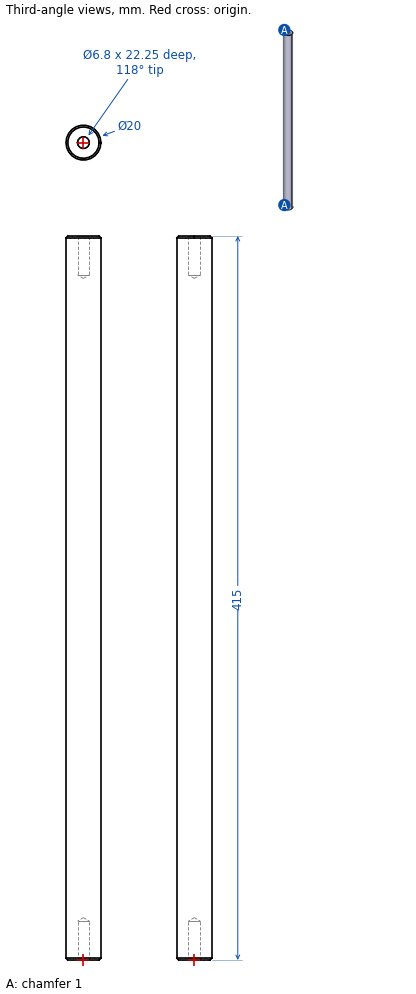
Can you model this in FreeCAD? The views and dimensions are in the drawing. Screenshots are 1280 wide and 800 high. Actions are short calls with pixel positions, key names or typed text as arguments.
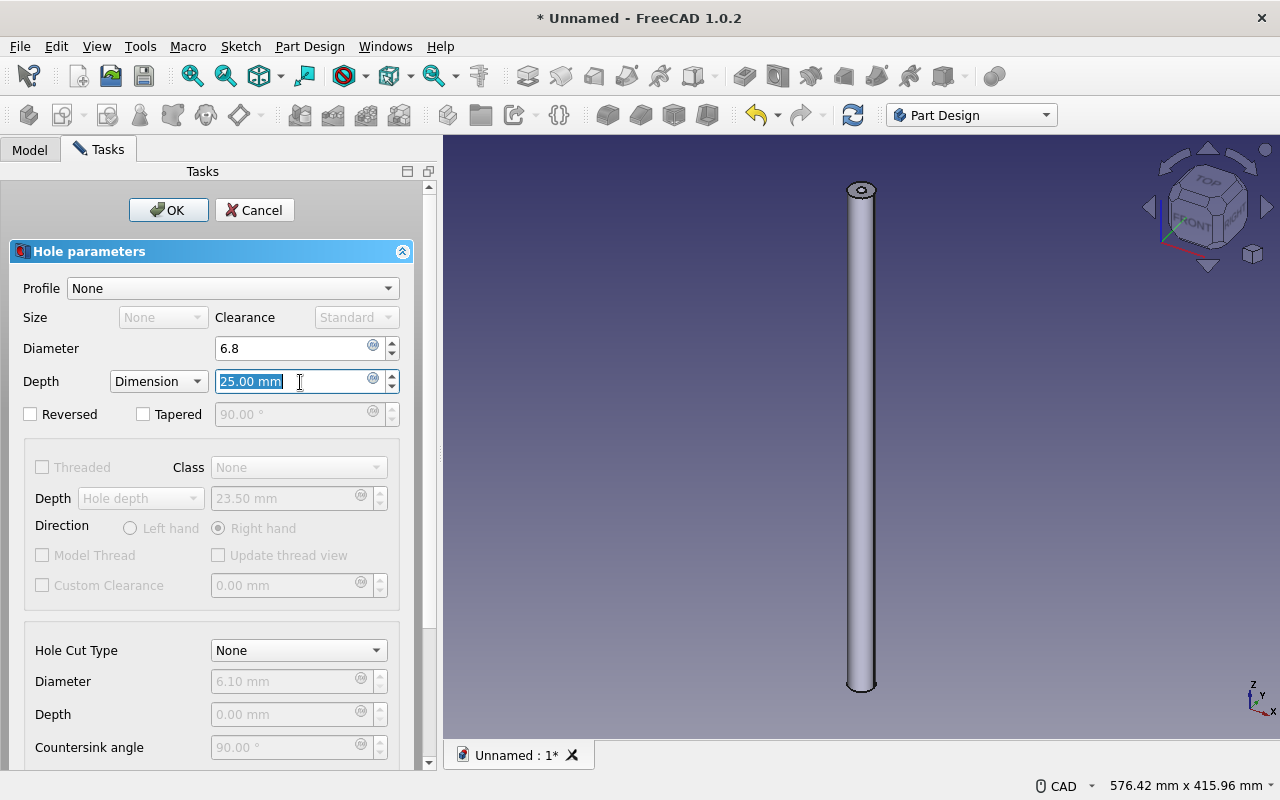
text(22.25)
key(Tab)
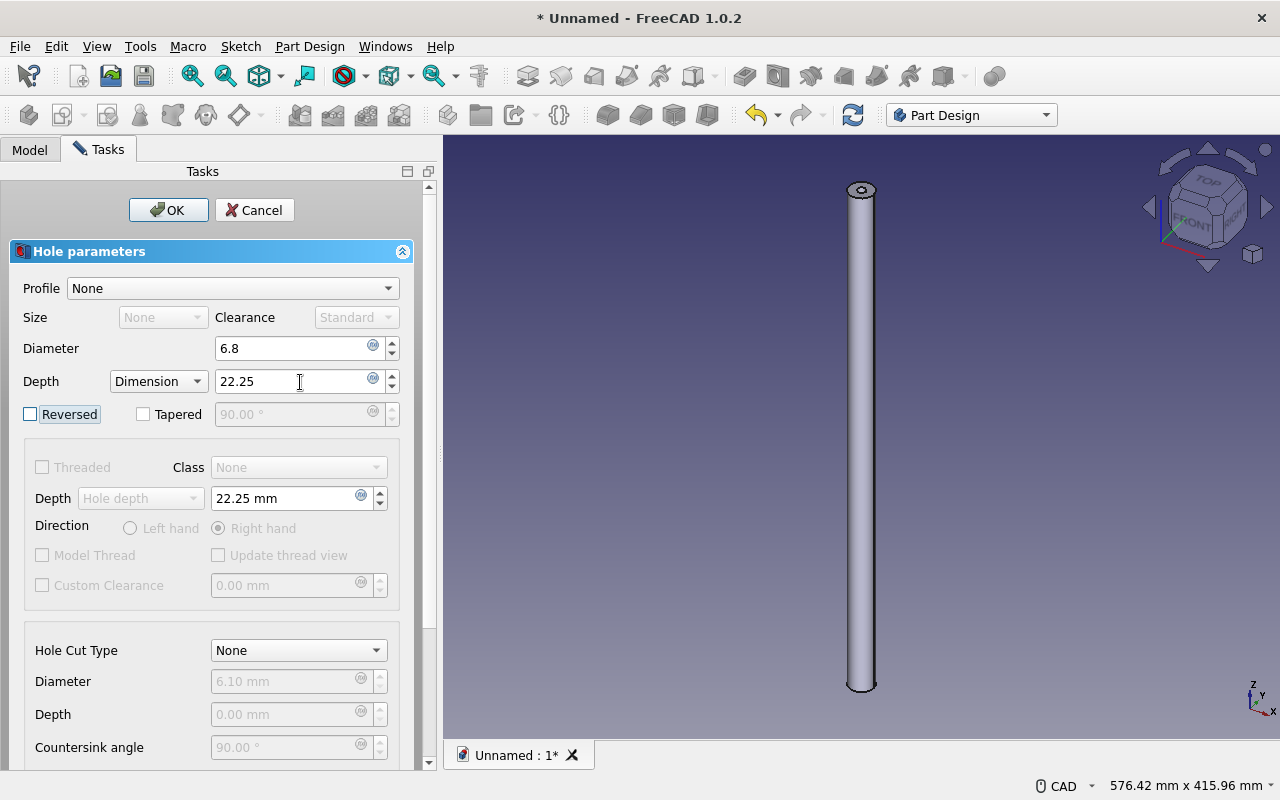
click(169, 210)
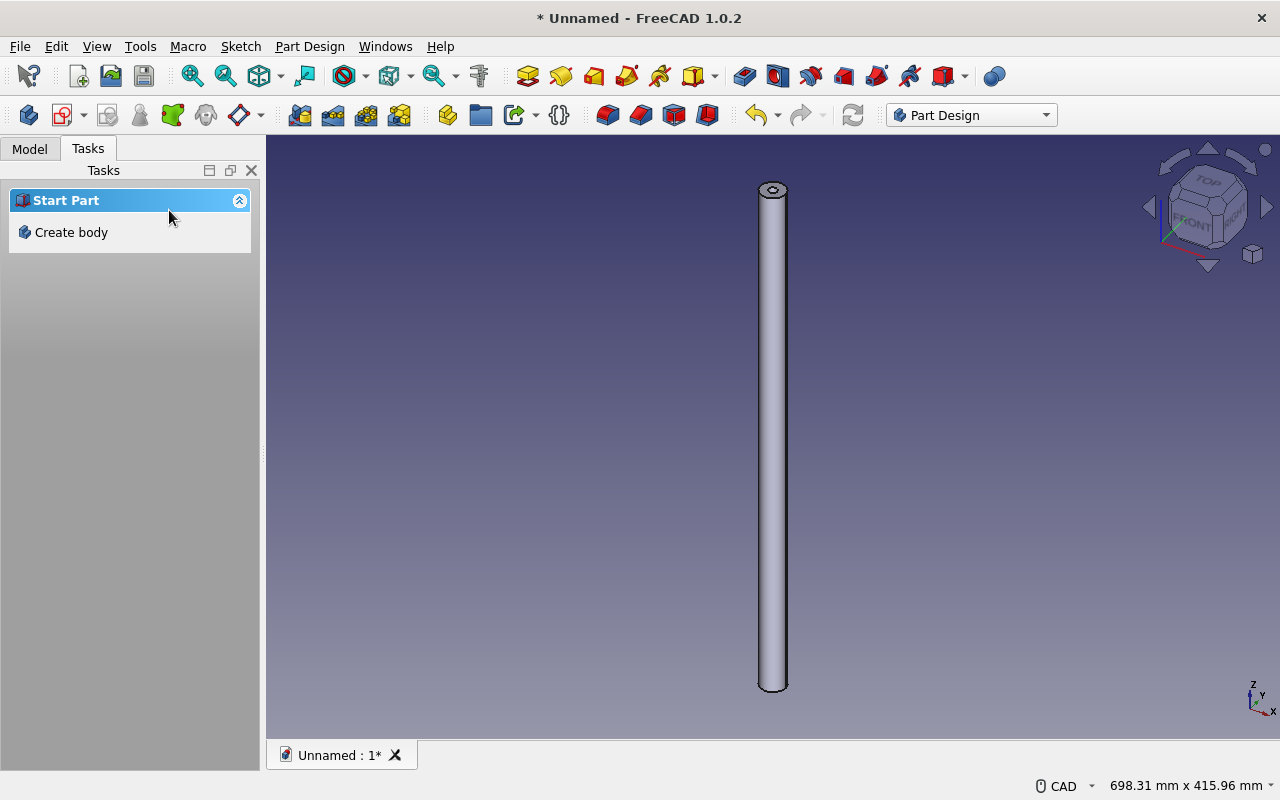
click(760, 185)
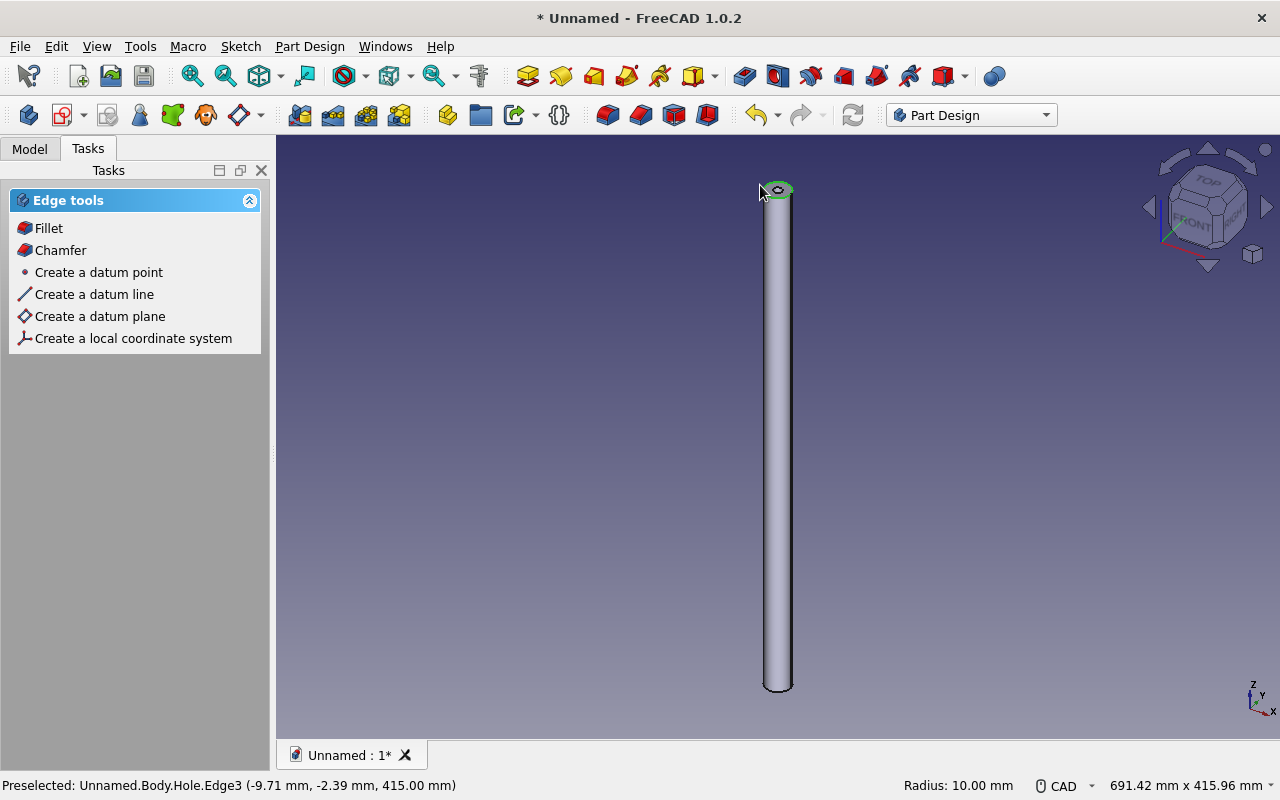
key(0)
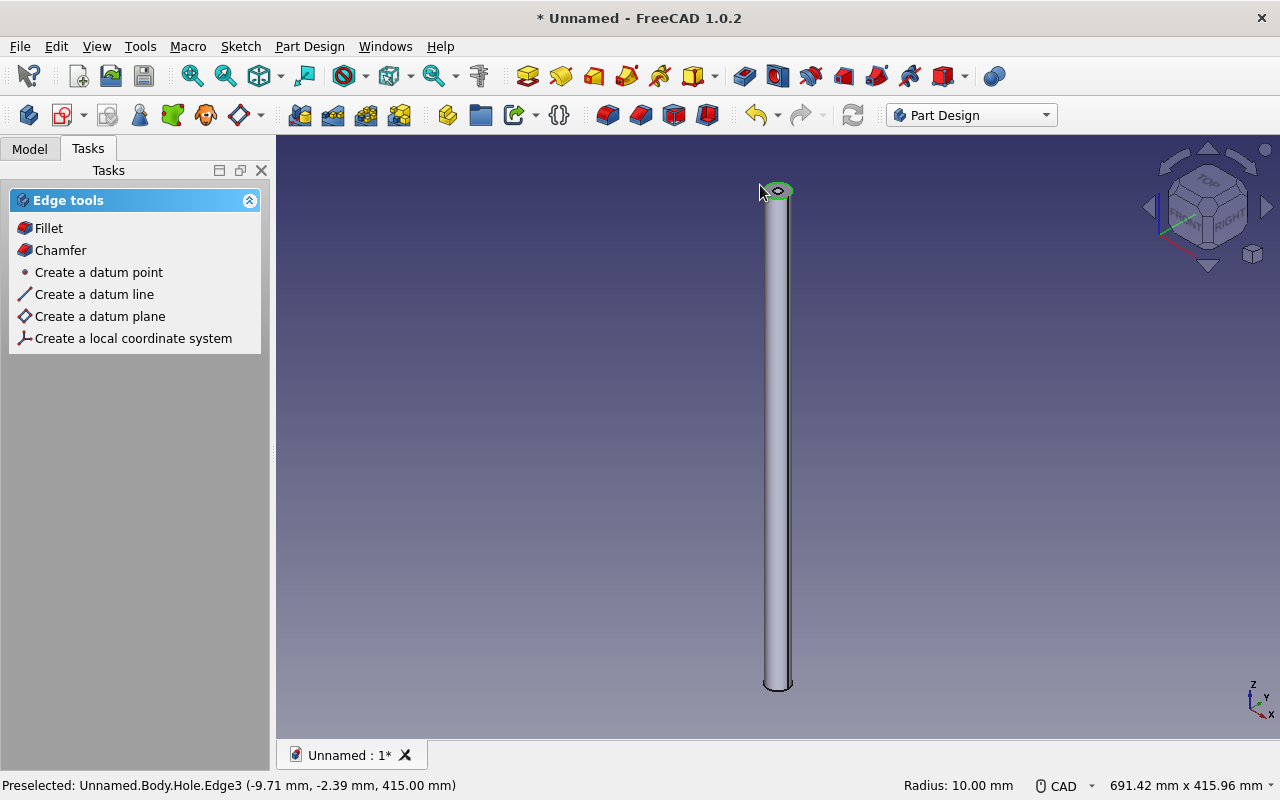
key(2)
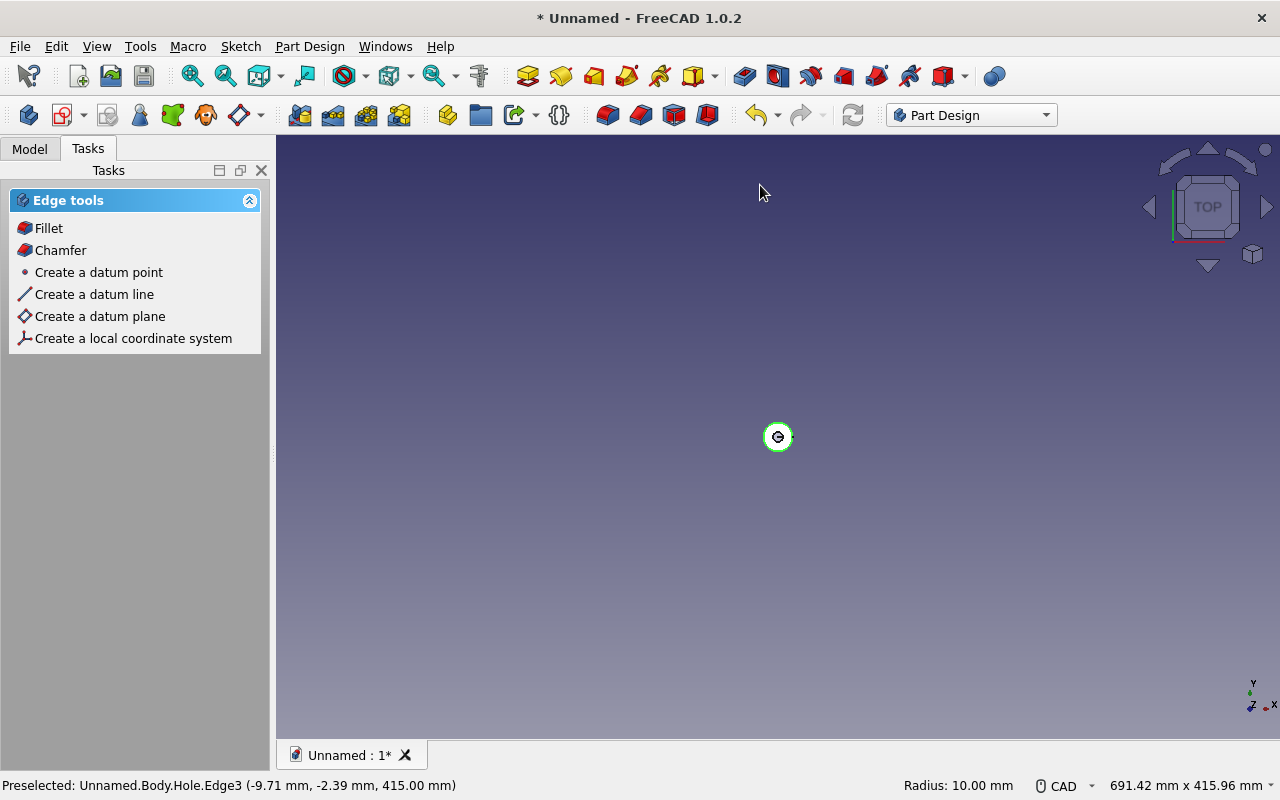
click(193, 76)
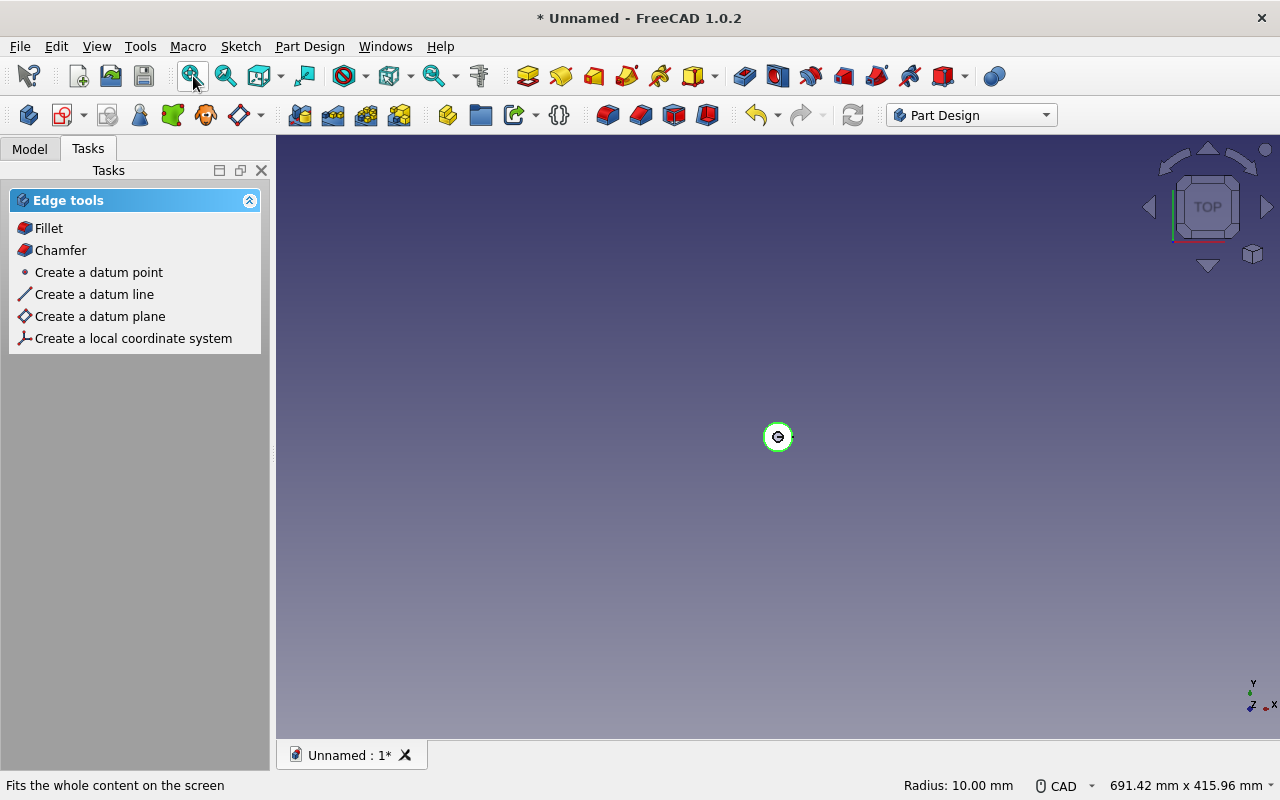
key(1)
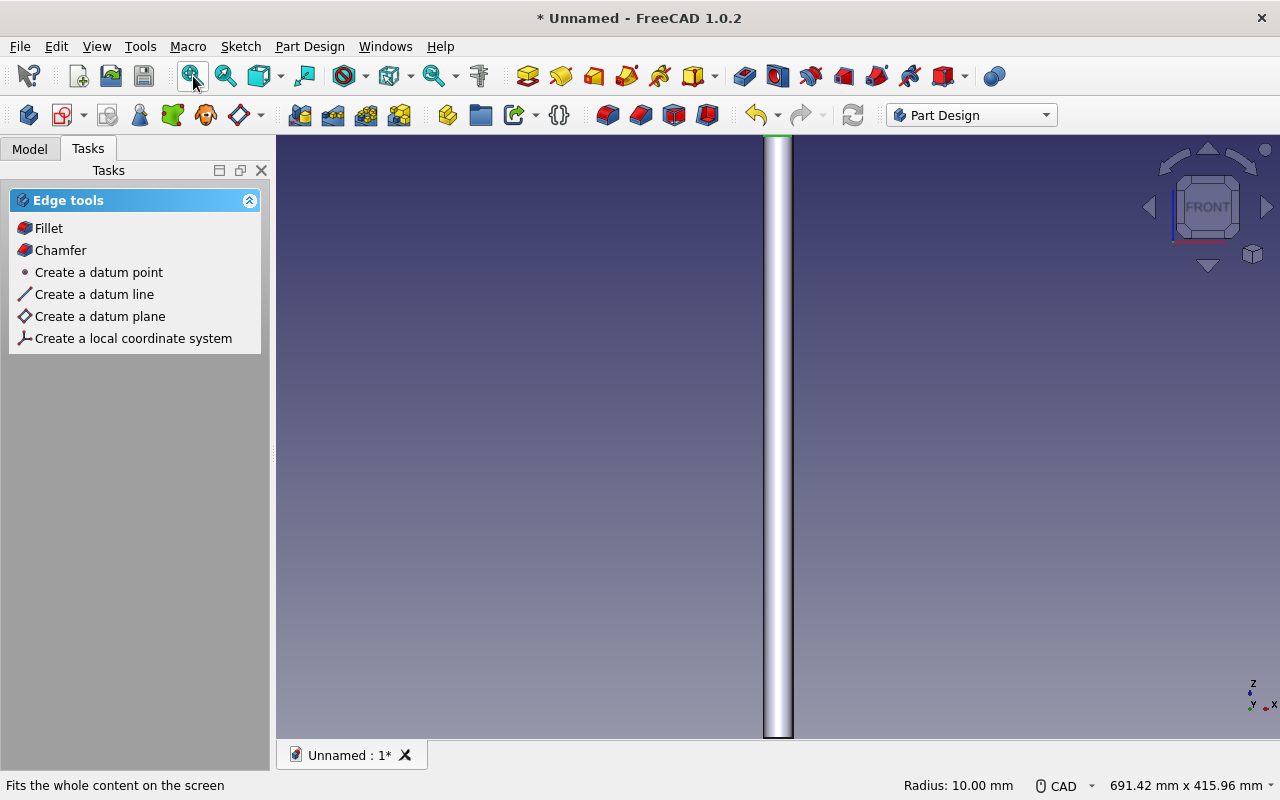
key(3)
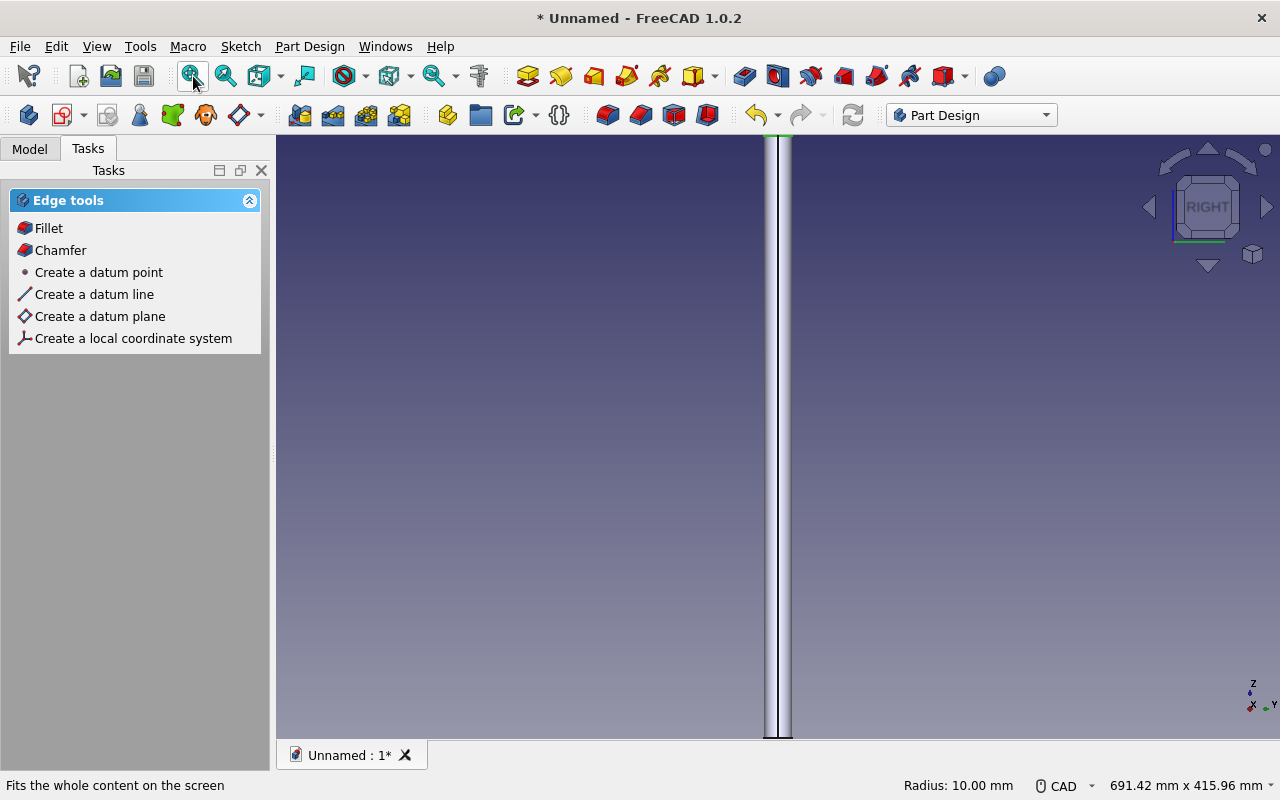
key(5)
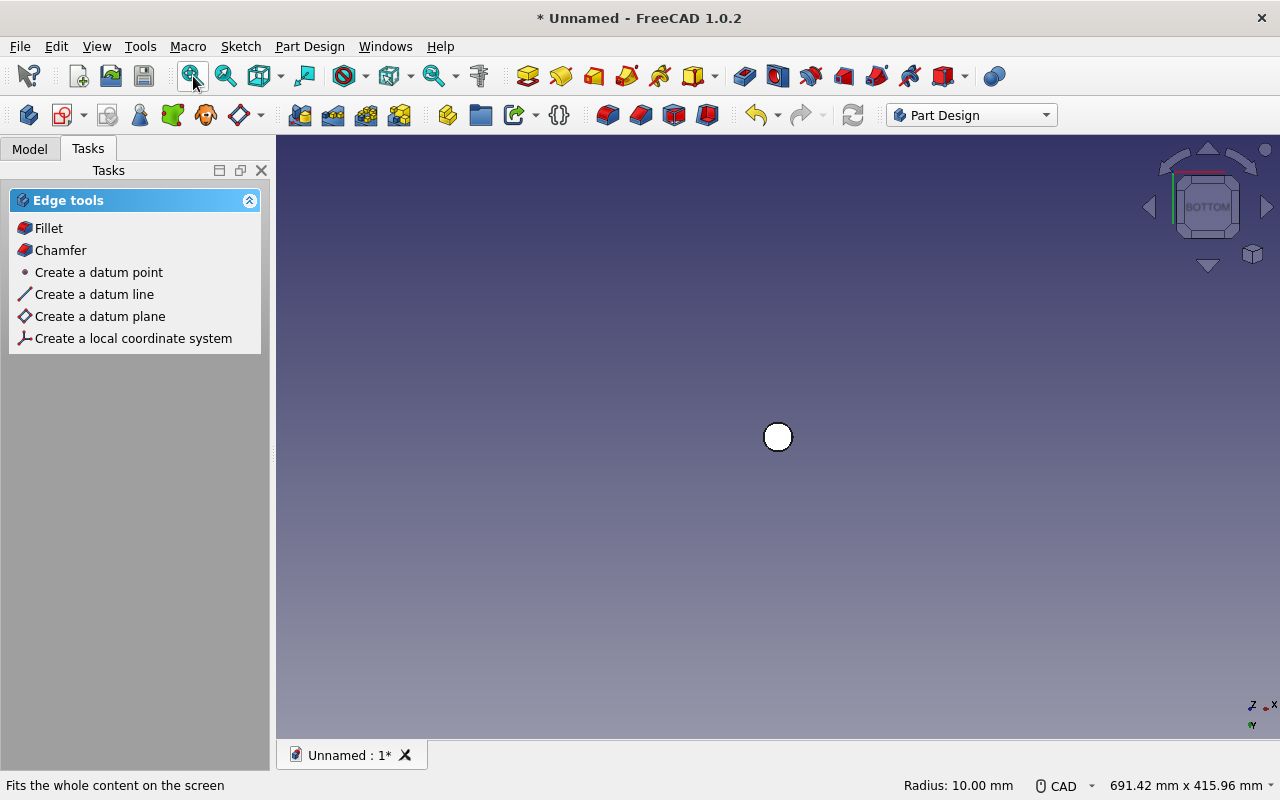
click(193, 76)